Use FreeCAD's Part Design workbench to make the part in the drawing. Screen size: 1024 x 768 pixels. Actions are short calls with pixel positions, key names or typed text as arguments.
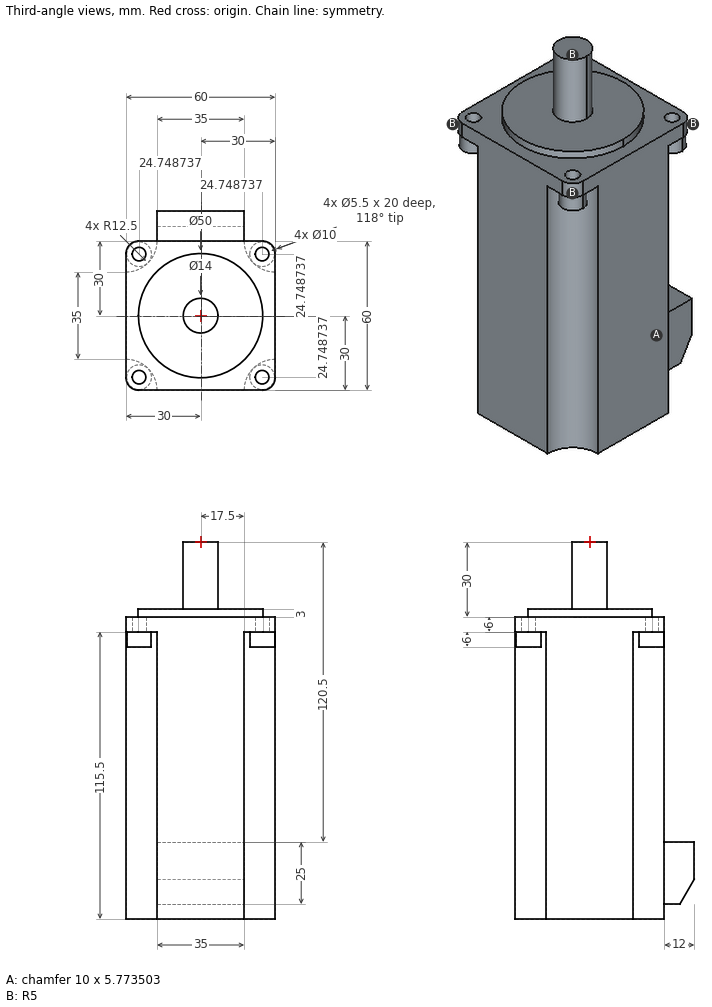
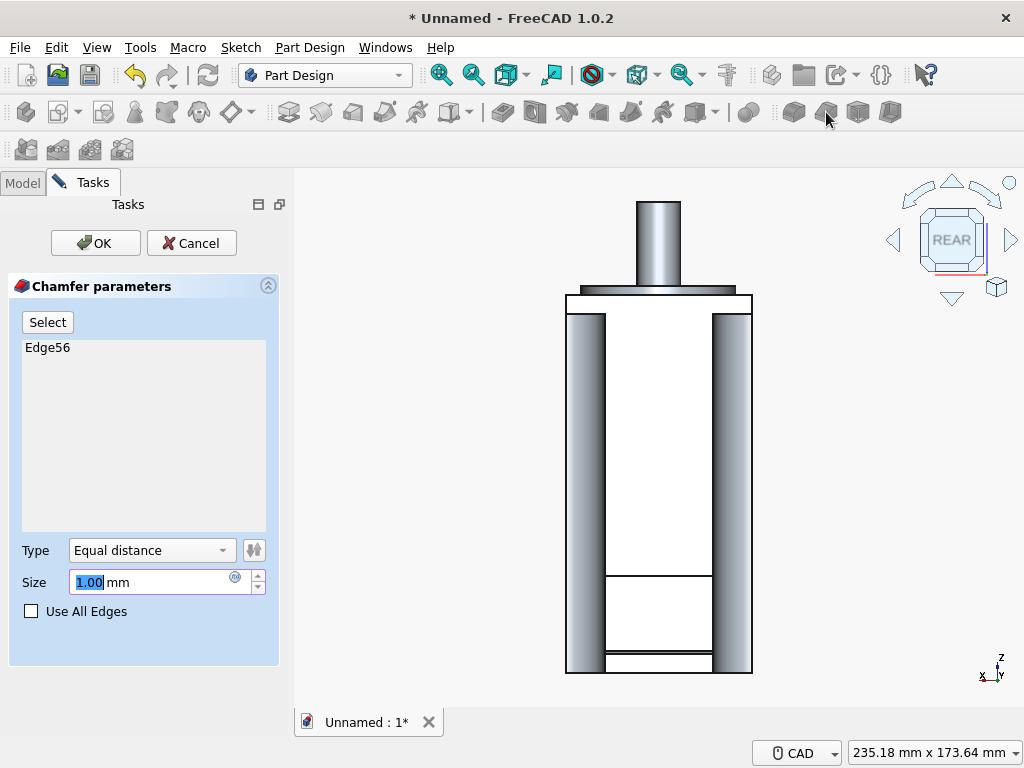
text(10)
key(Tab)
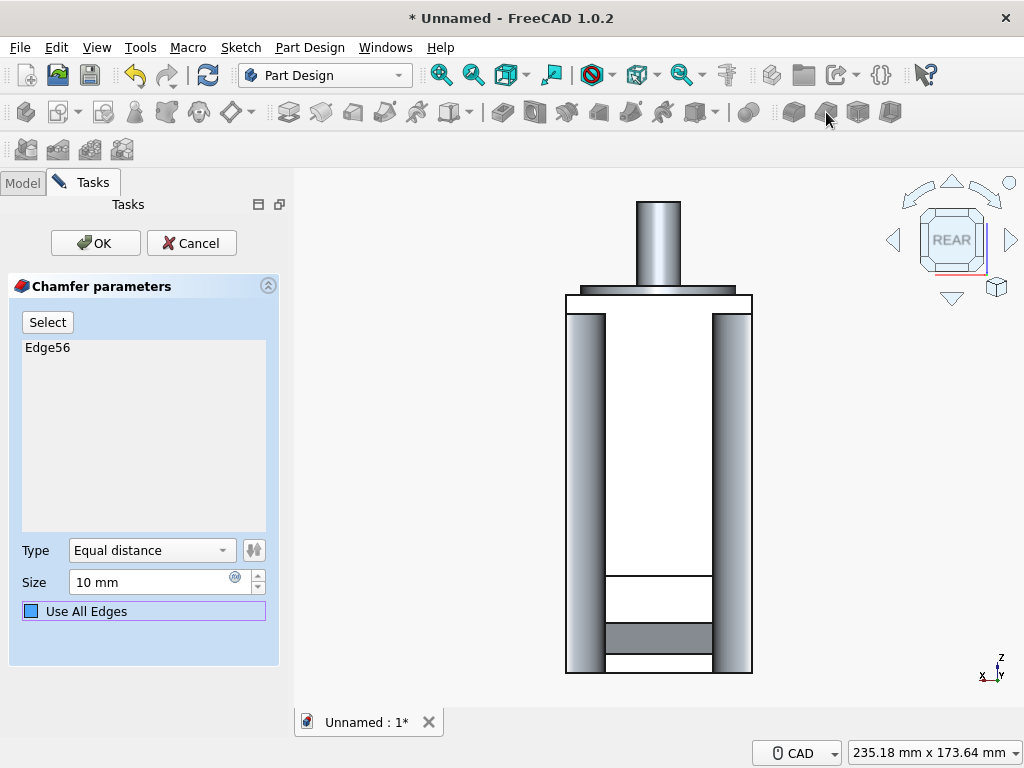
click(153, 550)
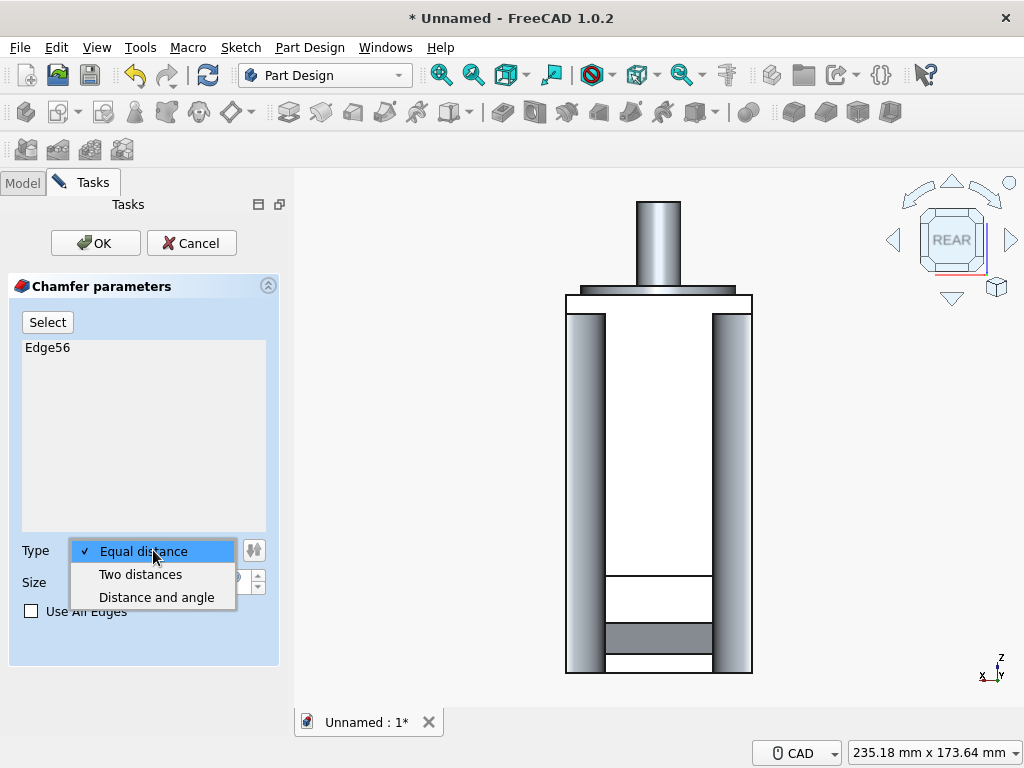
click(152, 574)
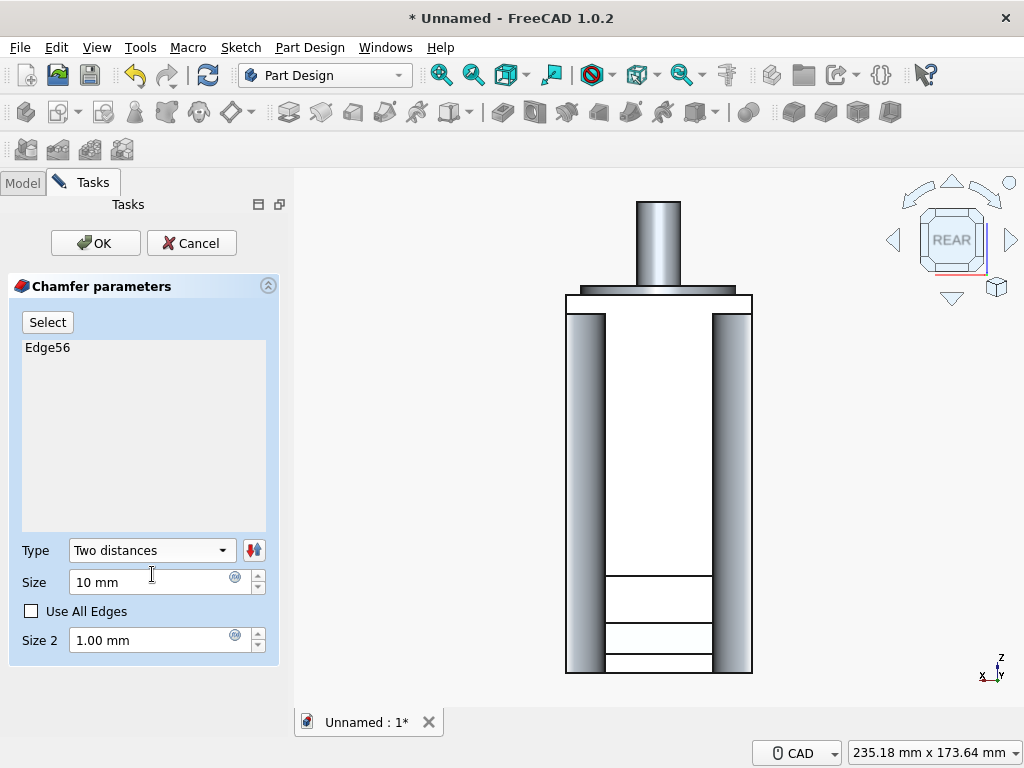
triple_click(160, 640)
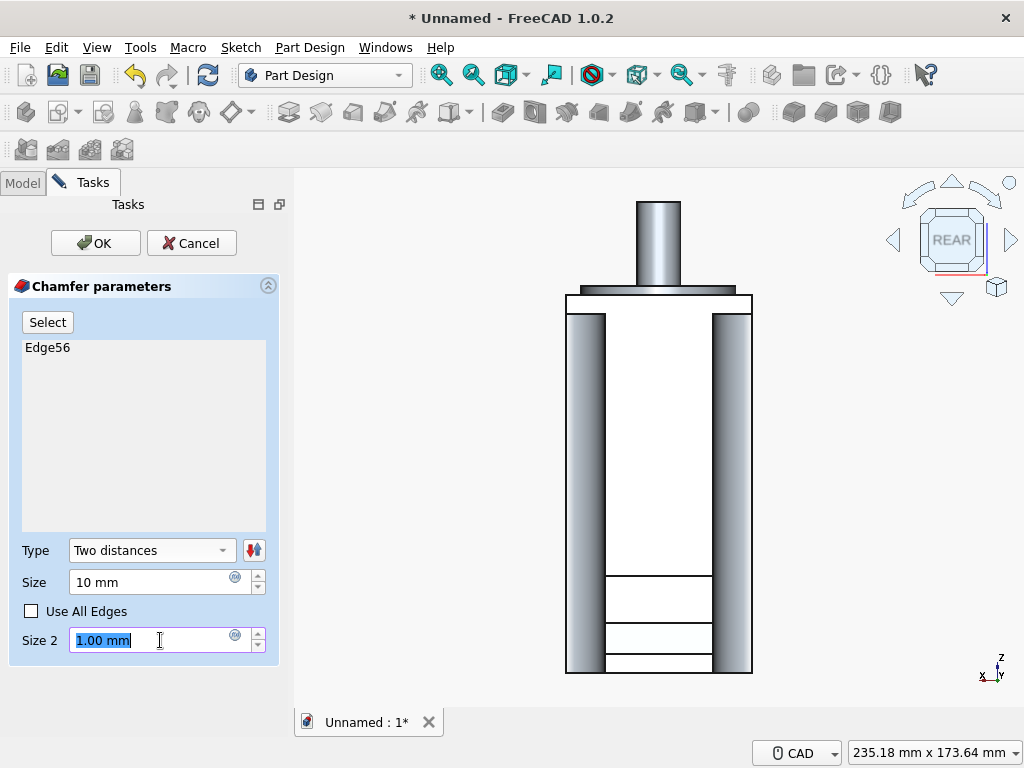
text(5.773503)
key(Tab)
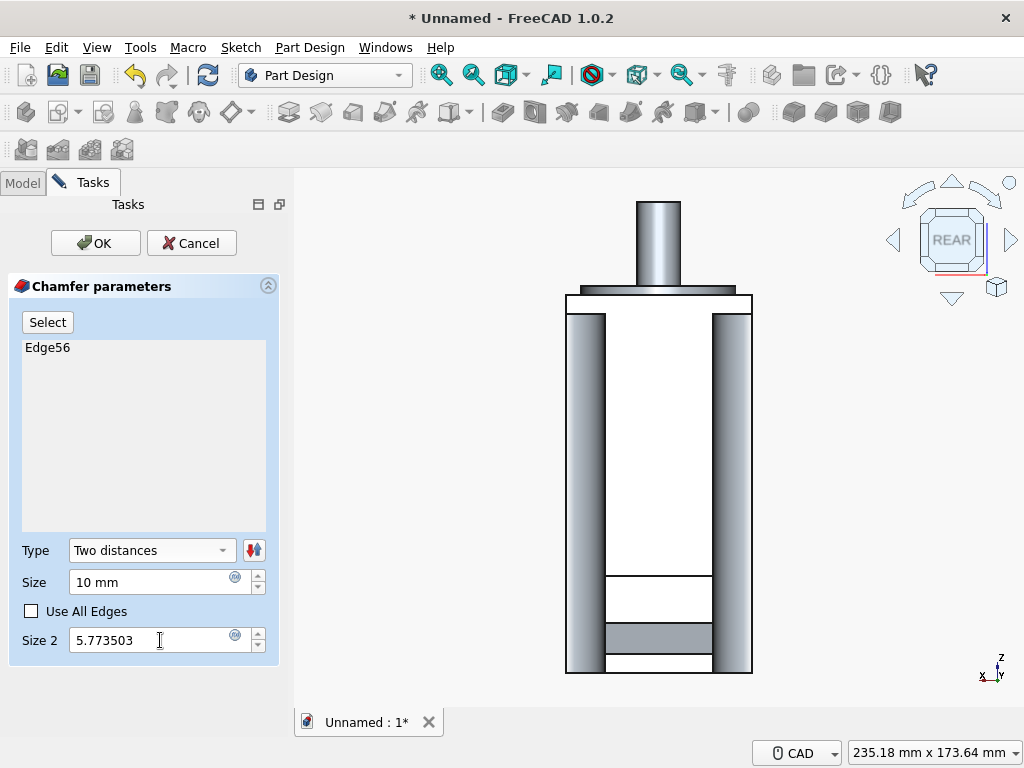
click(96, 243)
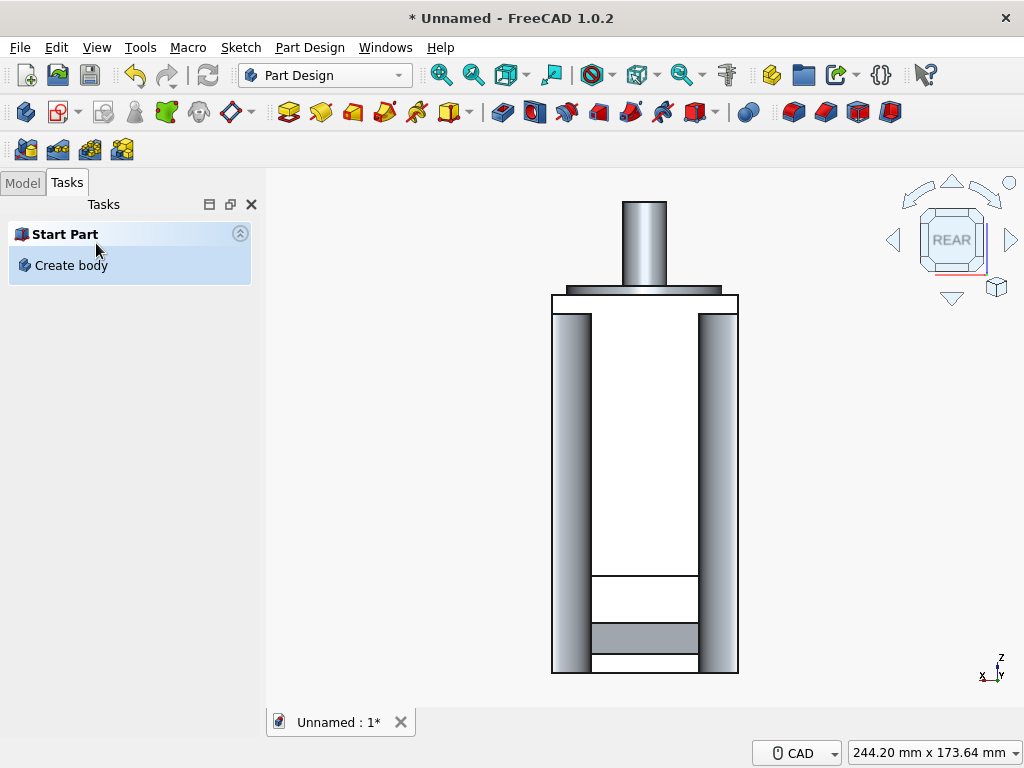
key(0)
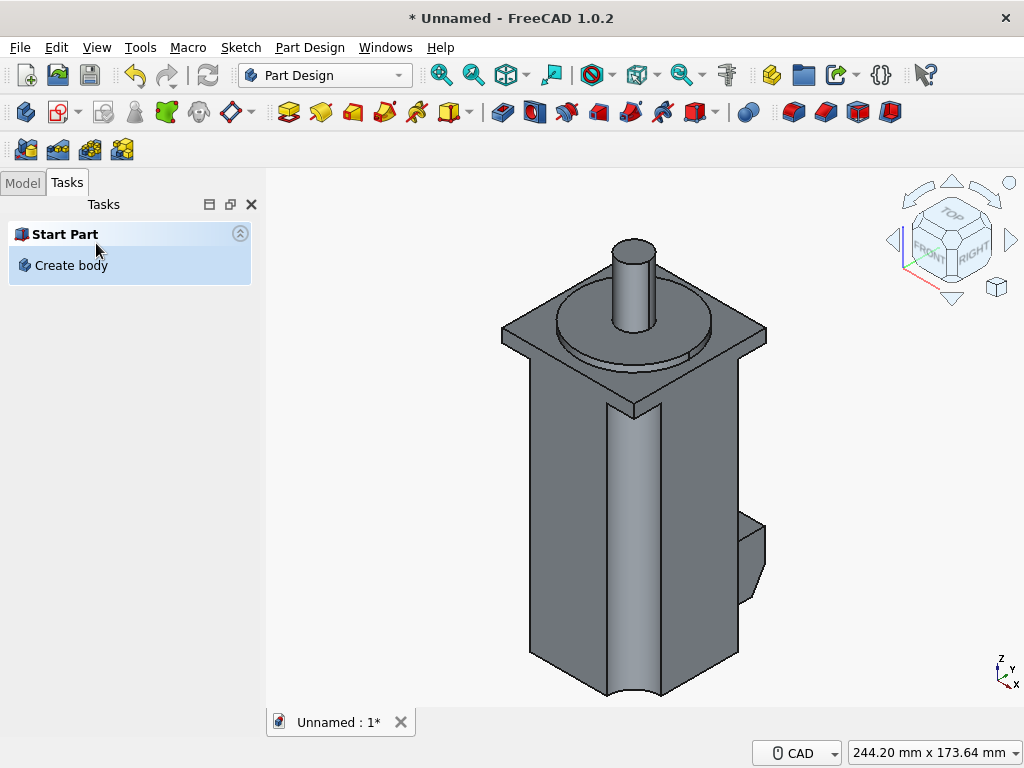
click(442, 76)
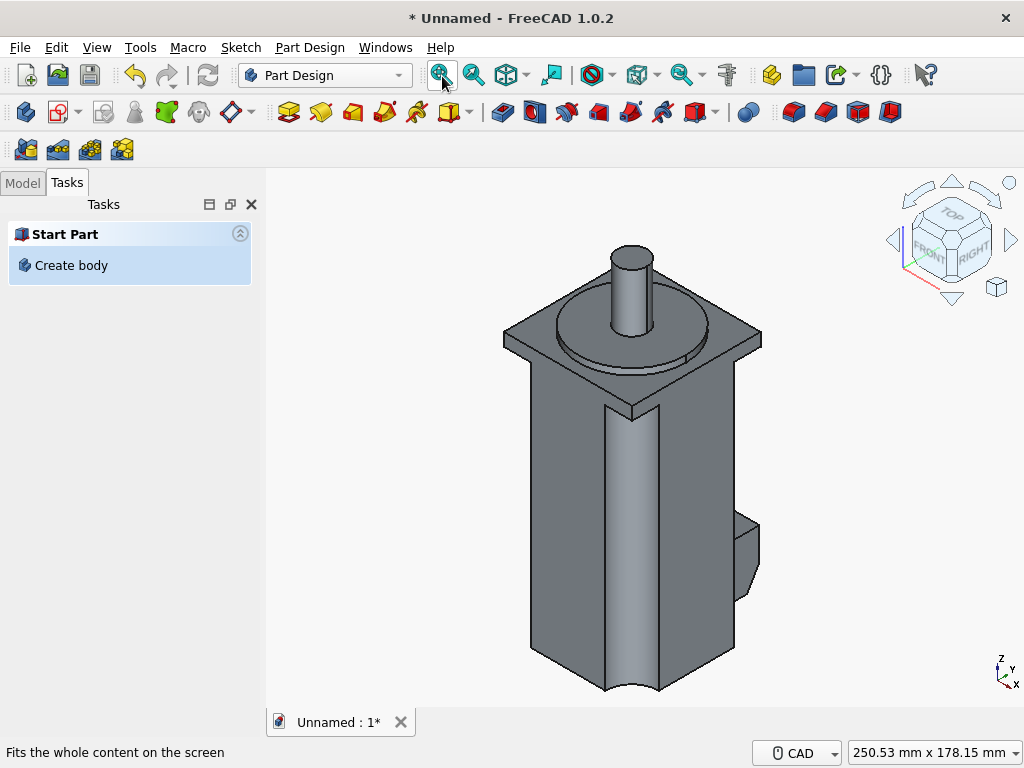
click(742, 331)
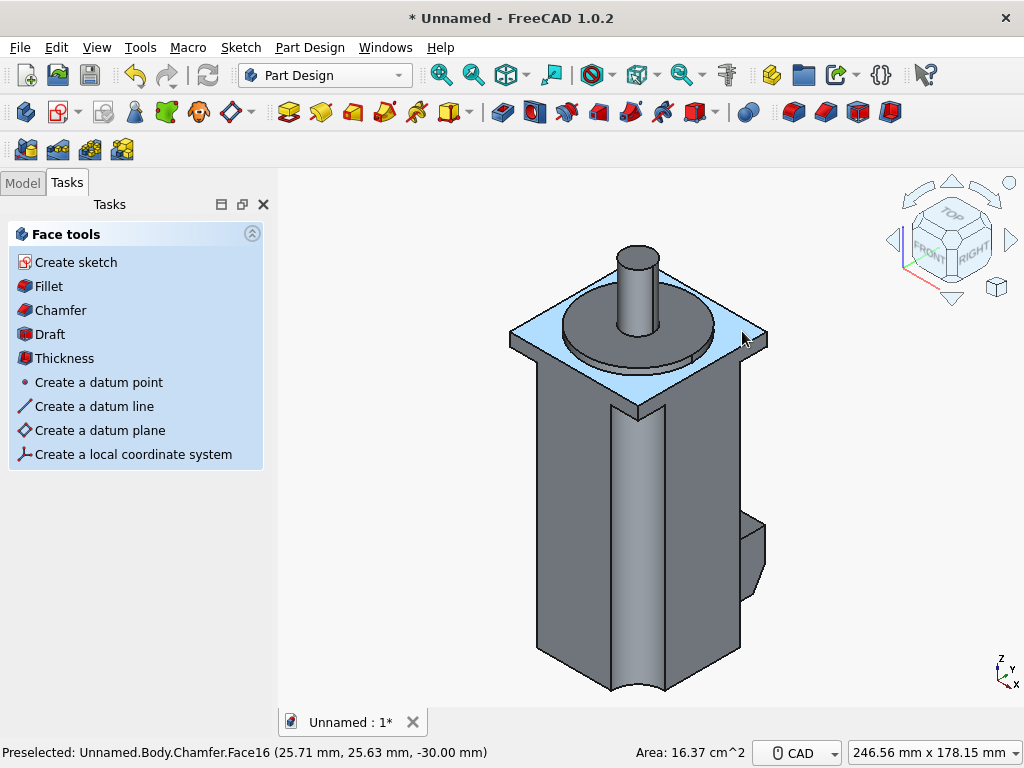
click(58, 112)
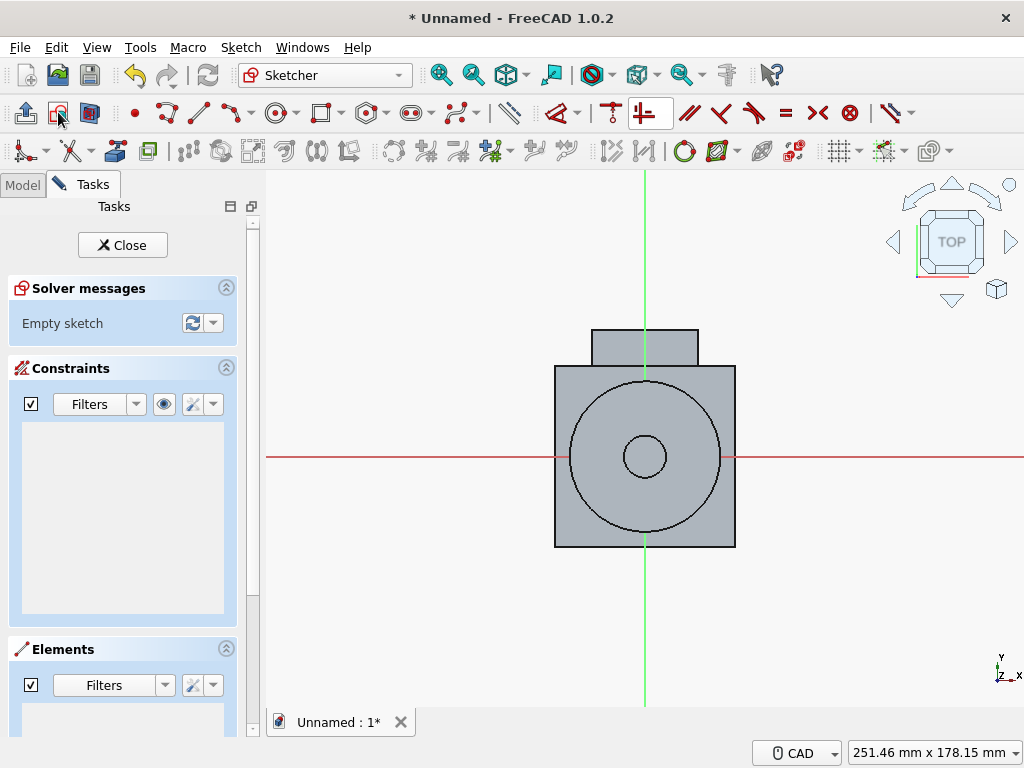
click(90, 114)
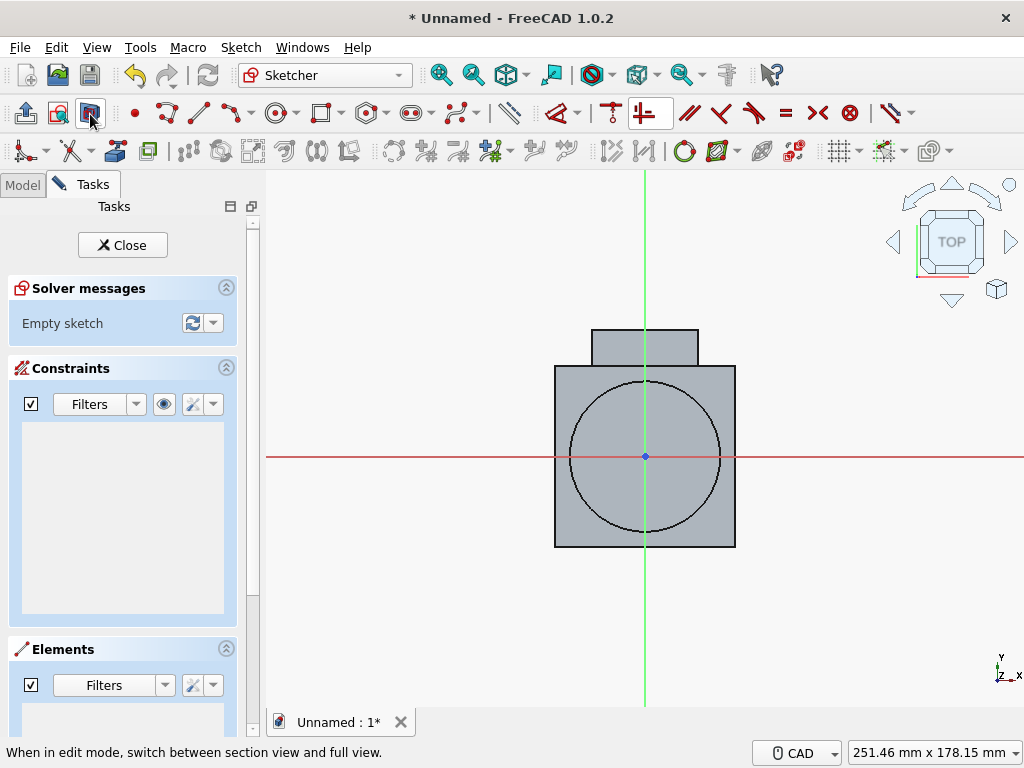
scroll(701, 471, up, 4)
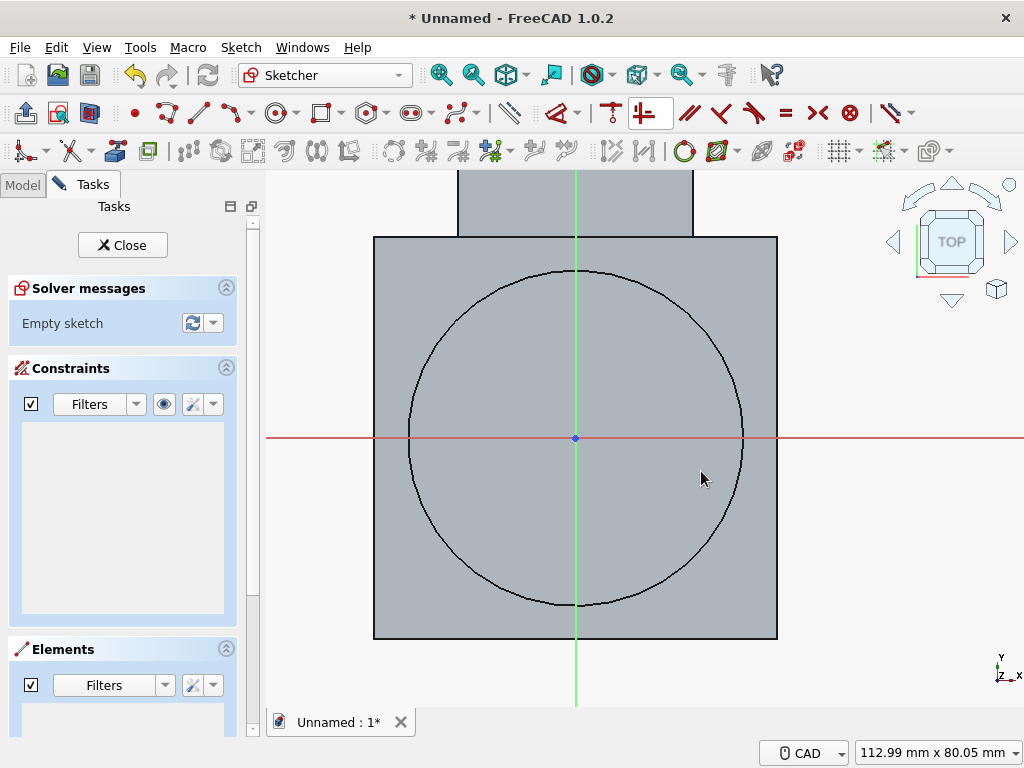
click(276, 114)